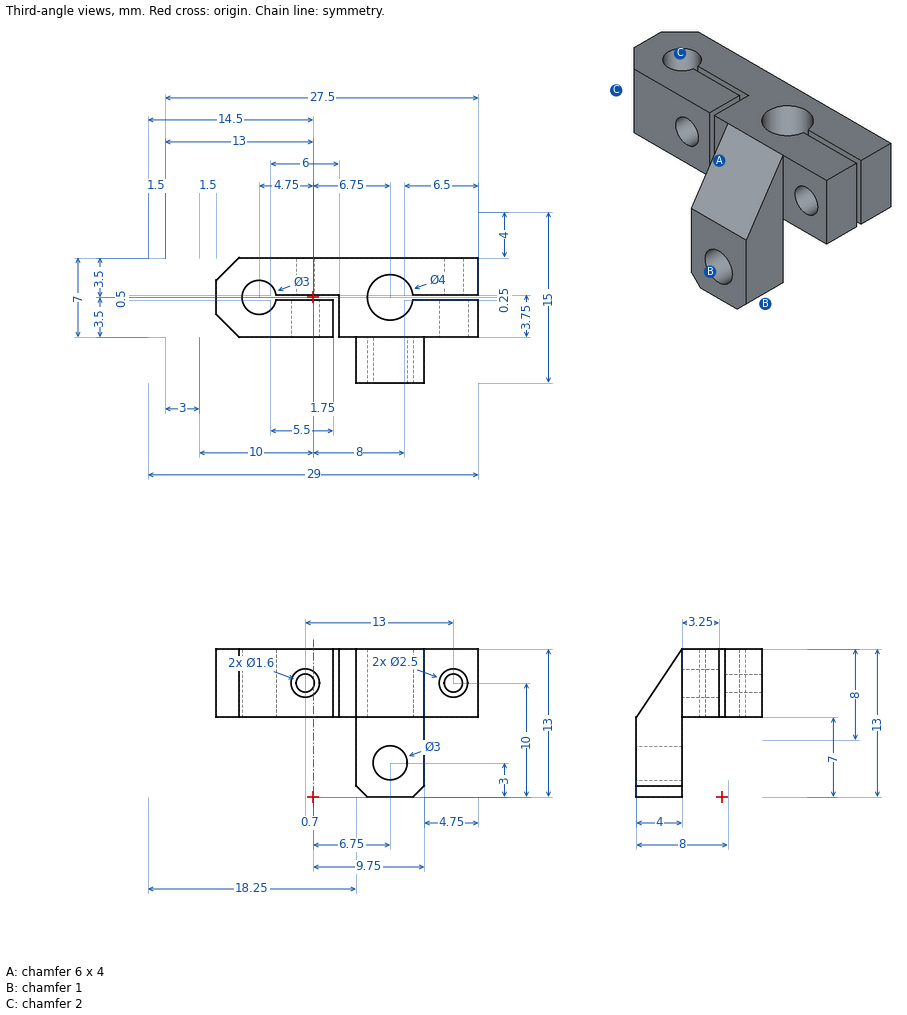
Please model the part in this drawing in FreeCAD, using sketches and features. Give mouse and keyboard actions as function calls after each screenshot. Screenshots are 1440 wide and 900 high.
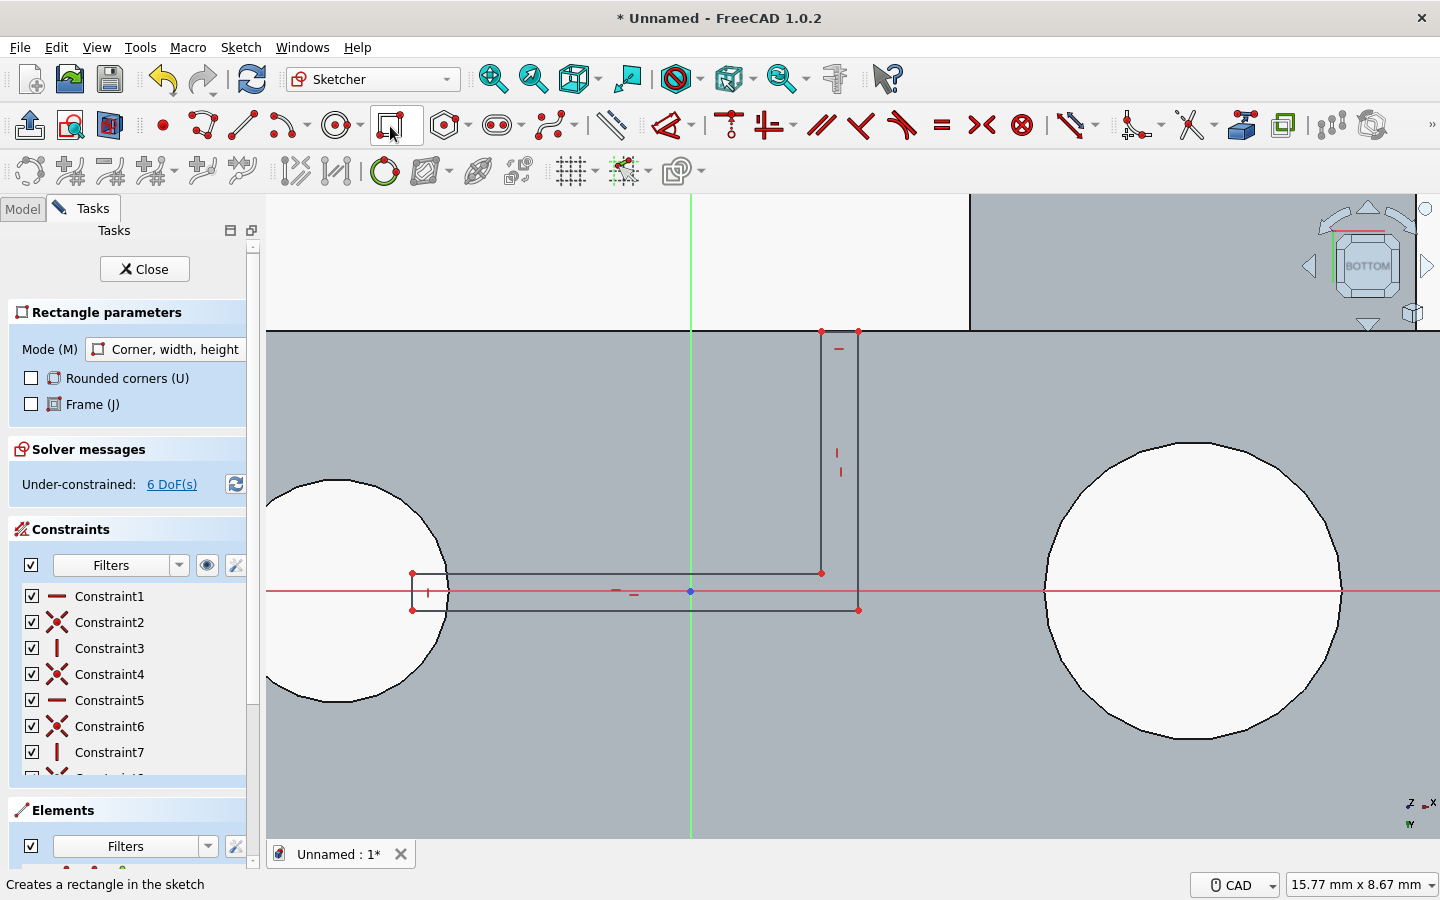
scroll(412, 573, down, 3)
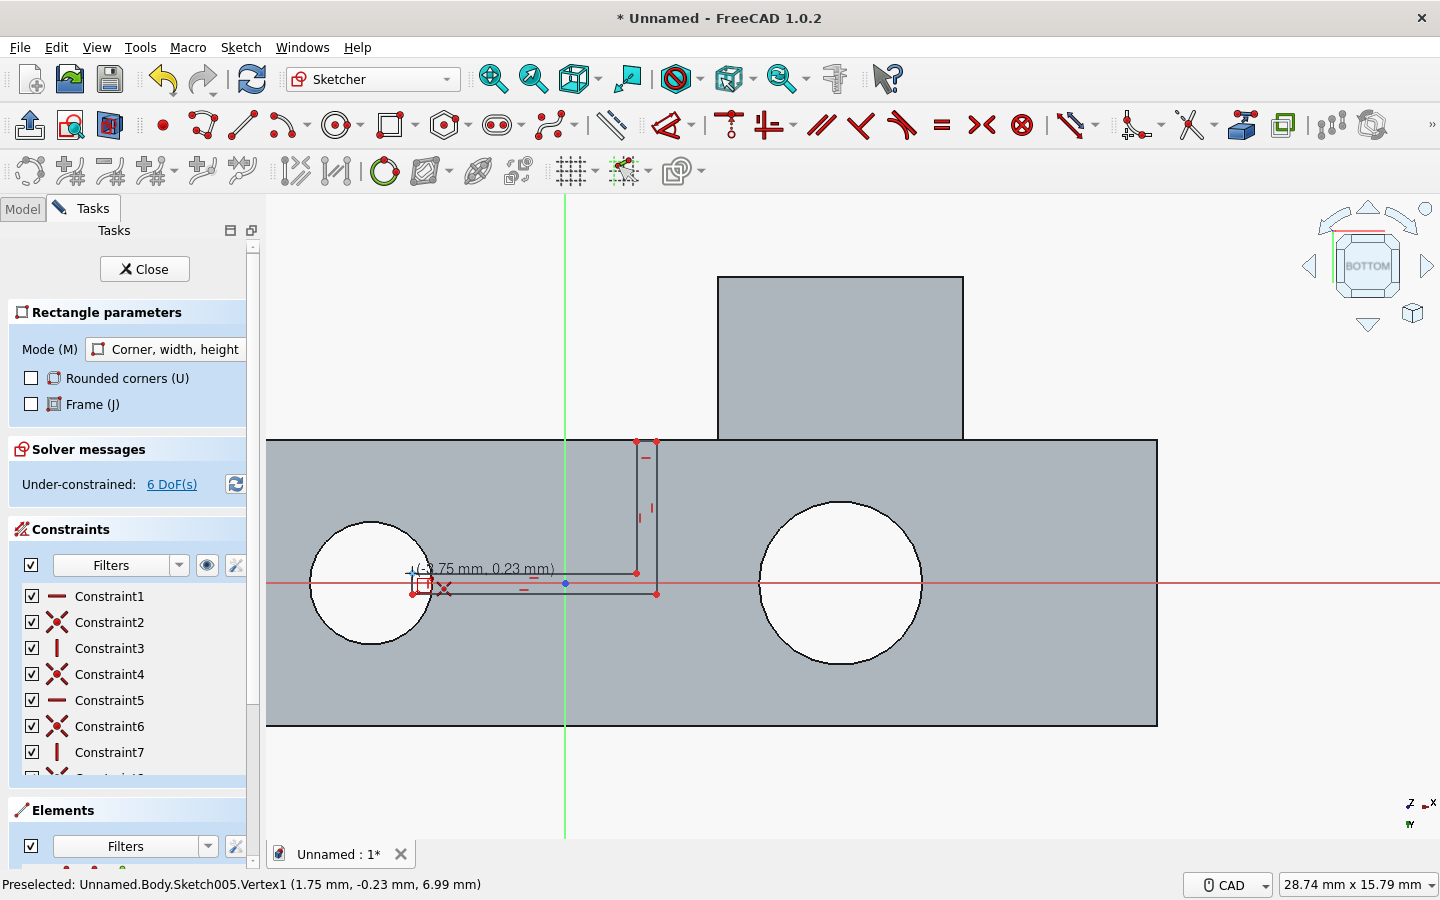
scroll(892, 573, up, 3)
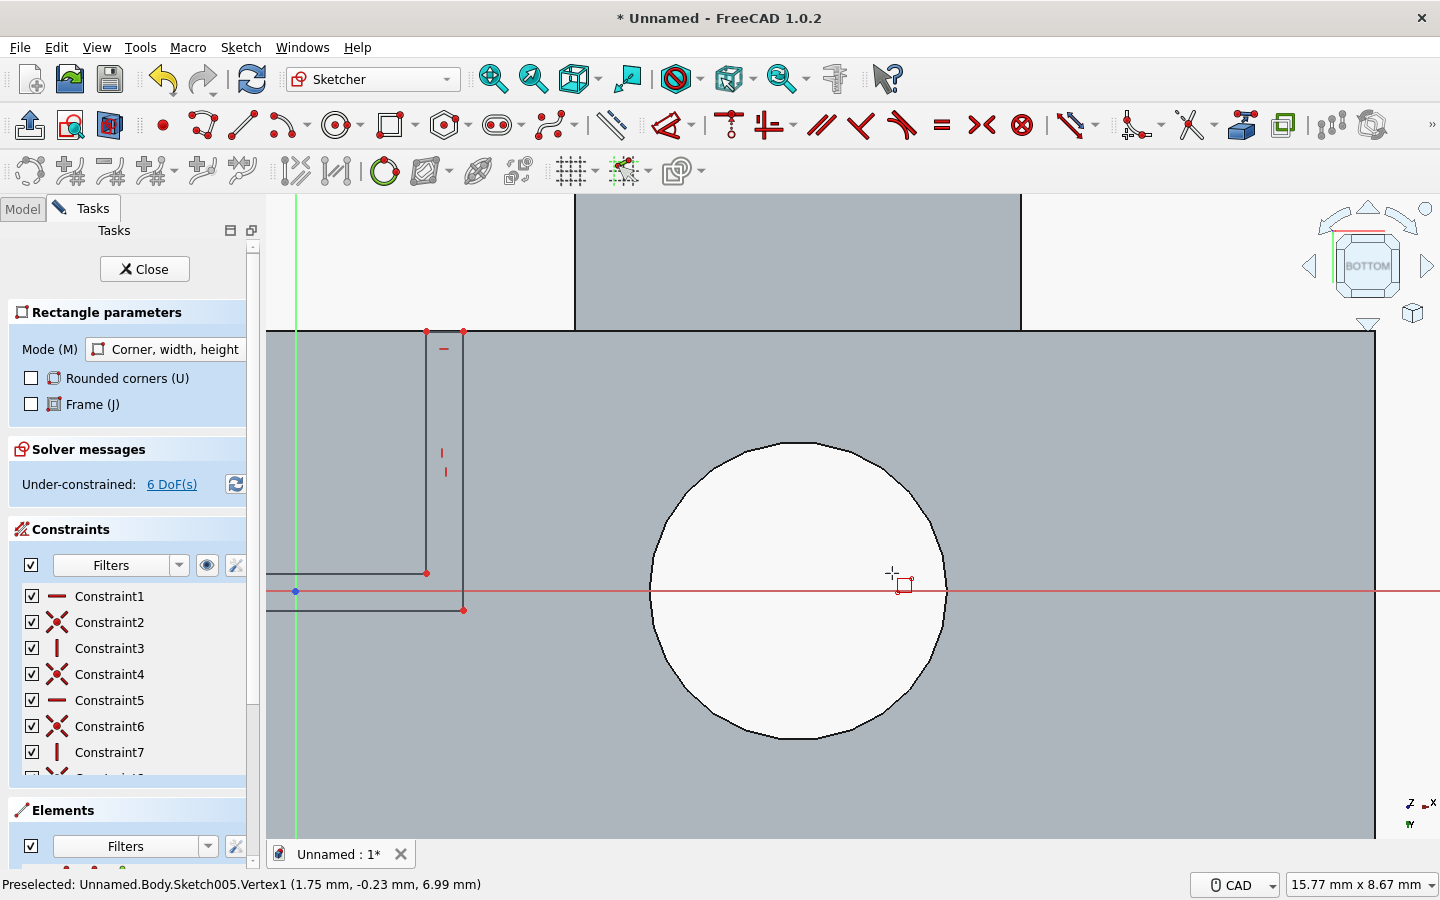
click(891, 573)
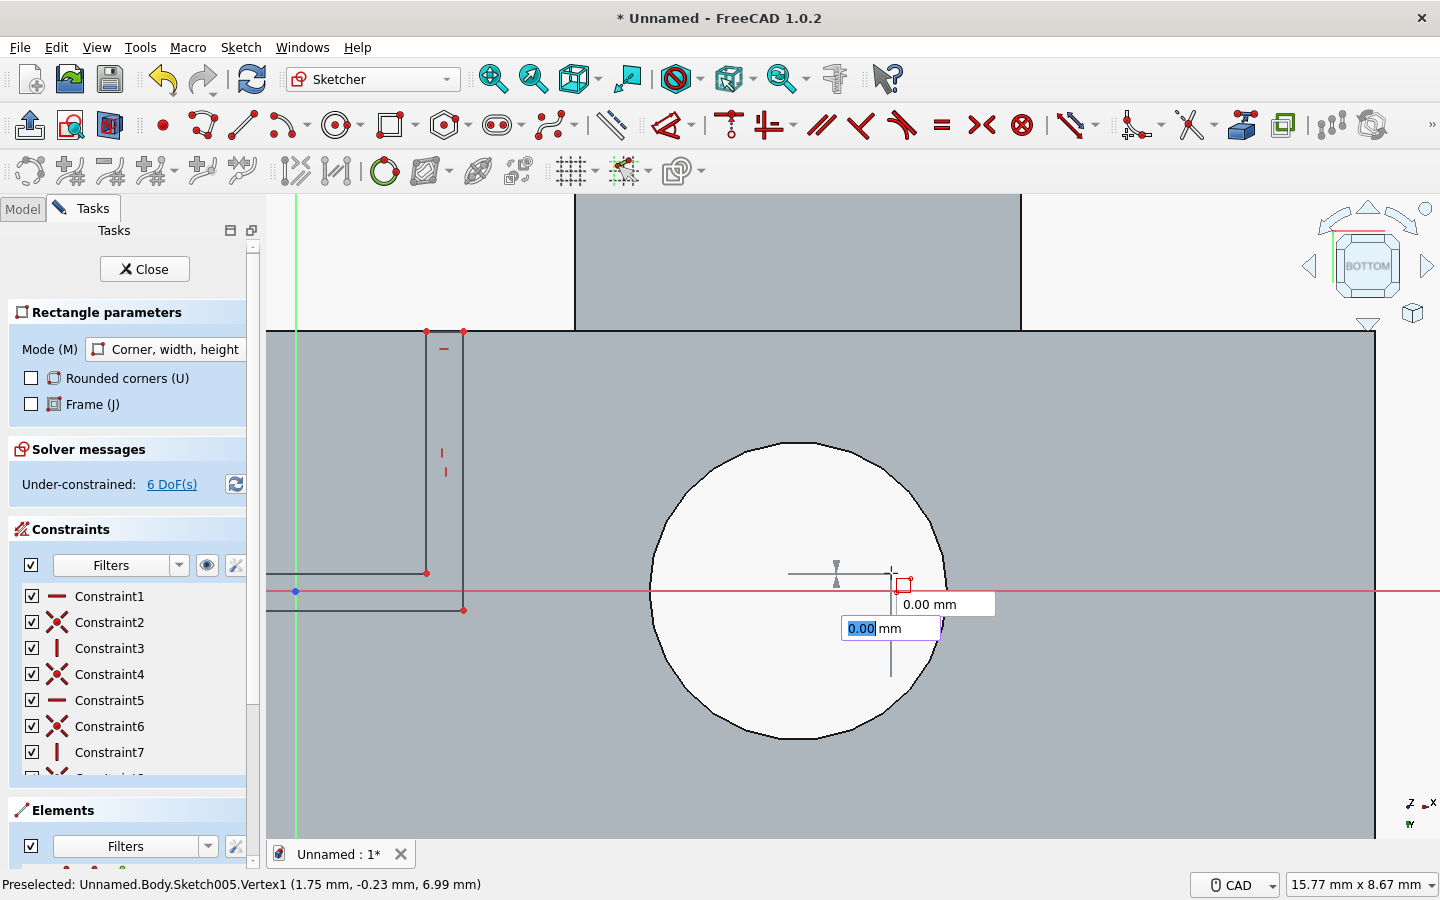
scroll(892, 573, down, 3)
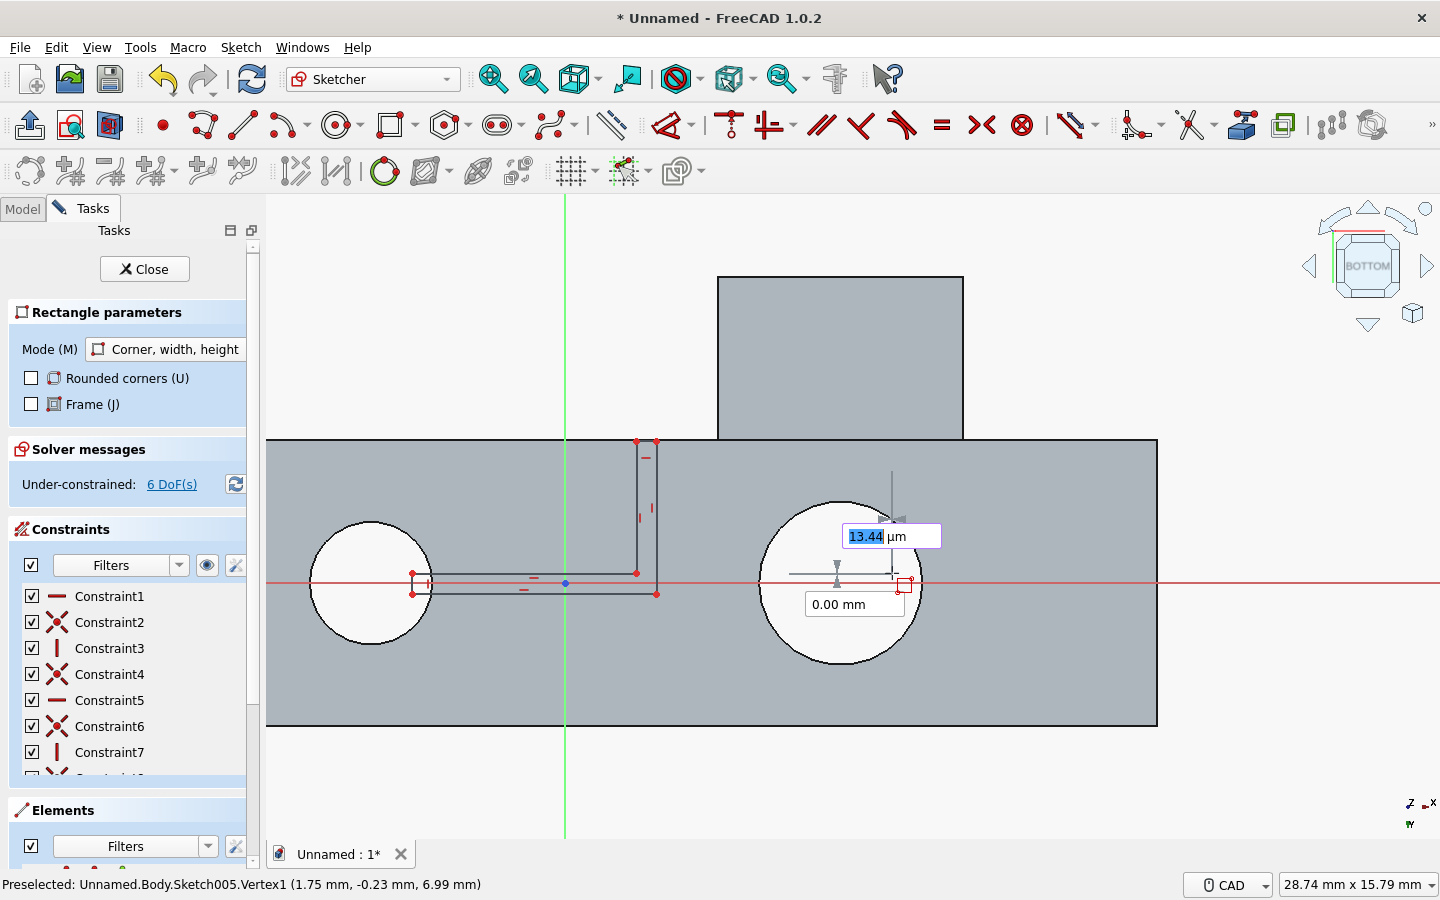
scroll(1157, 593, up, 3)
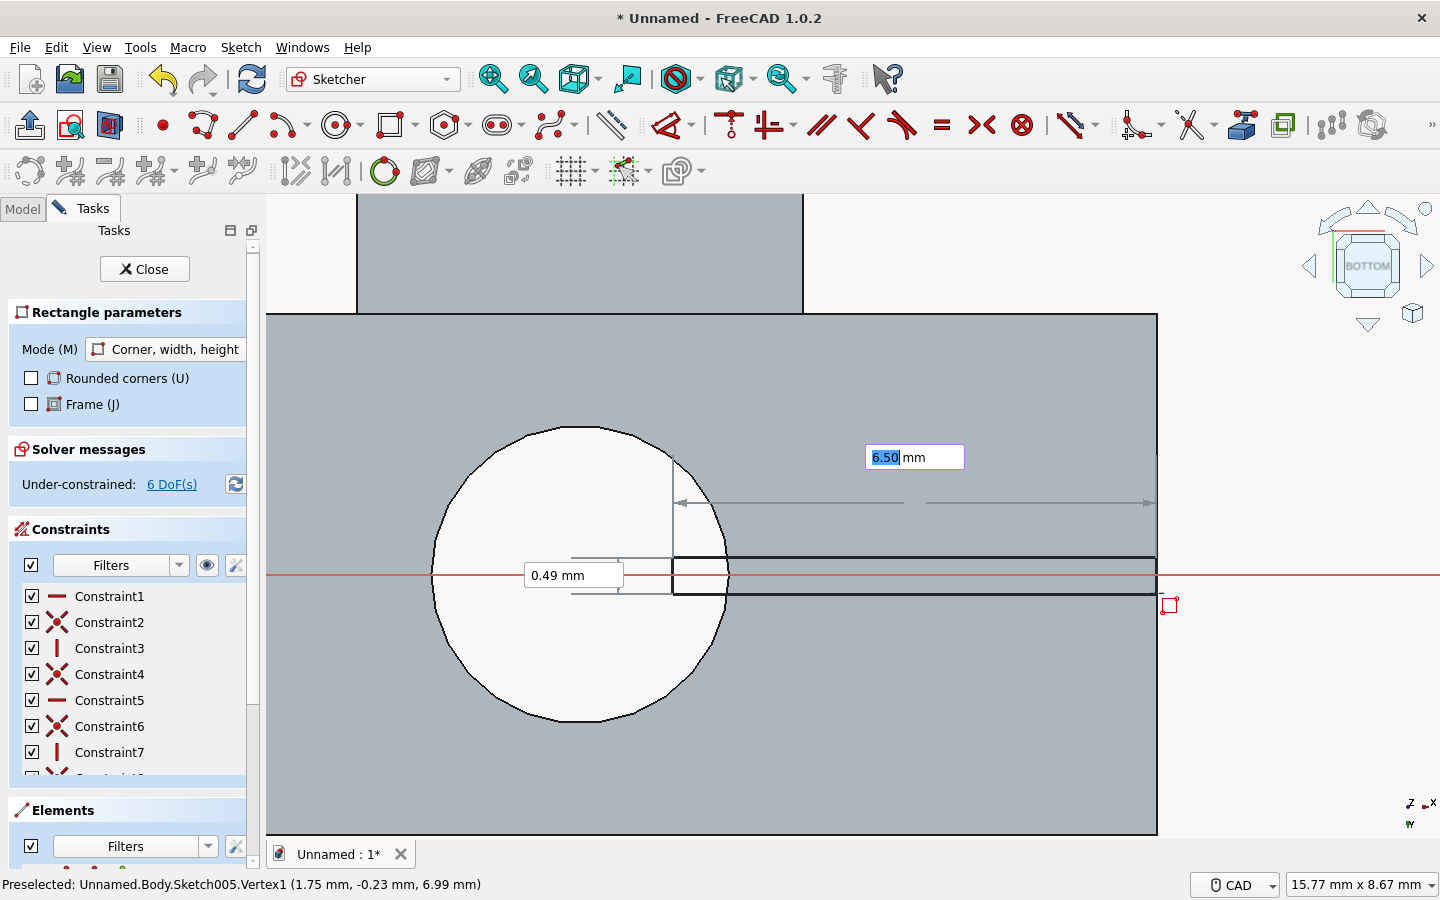
click(1157, 593)
key(Escape)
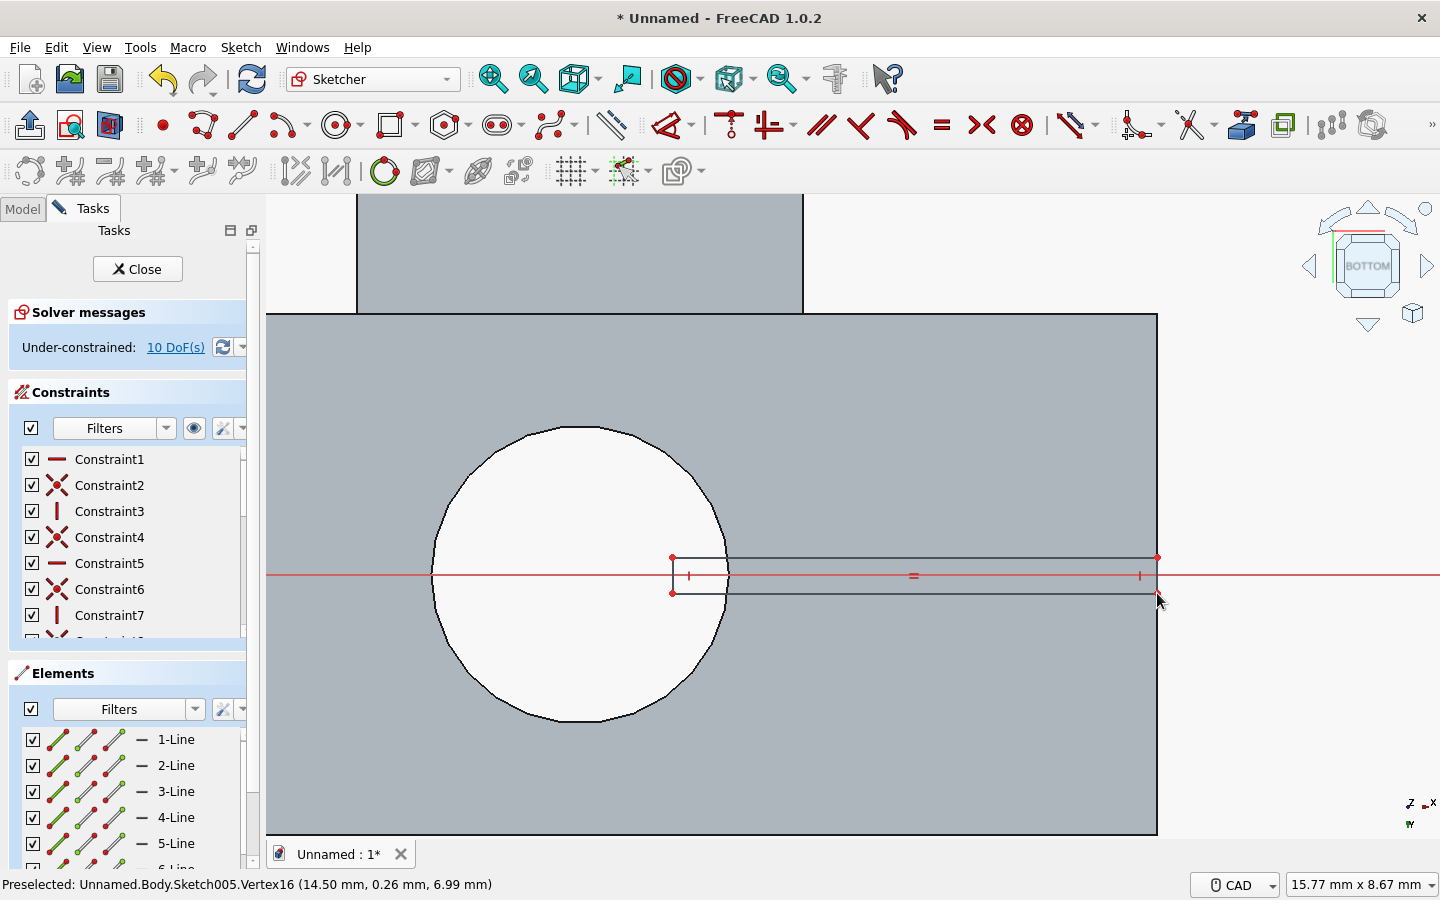
click(666, 126)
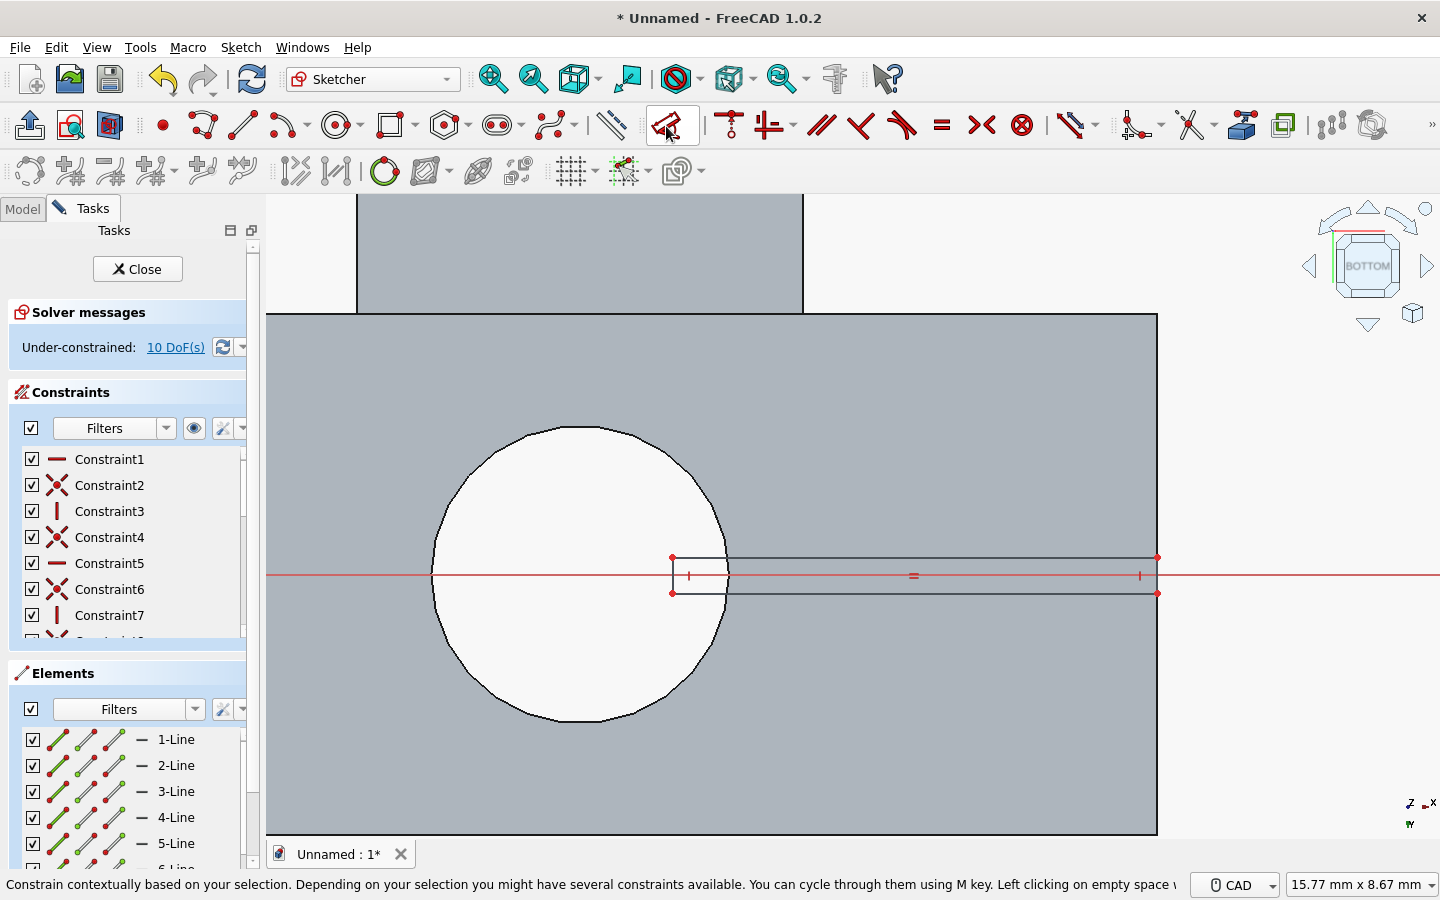
scroll(1158, 593, down, 3)